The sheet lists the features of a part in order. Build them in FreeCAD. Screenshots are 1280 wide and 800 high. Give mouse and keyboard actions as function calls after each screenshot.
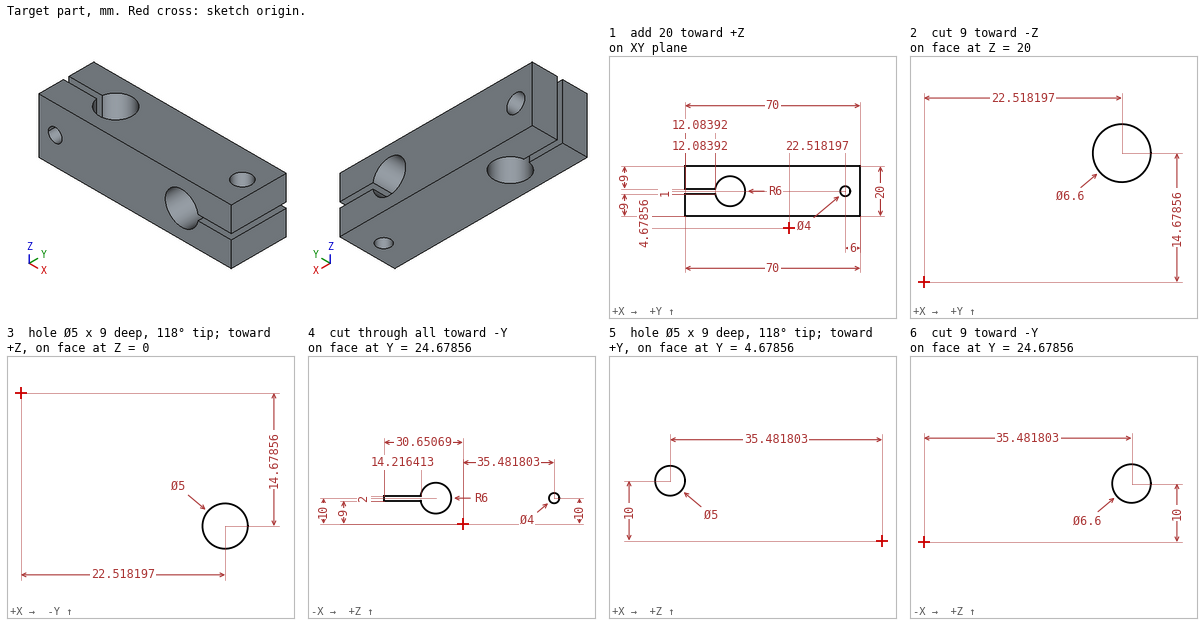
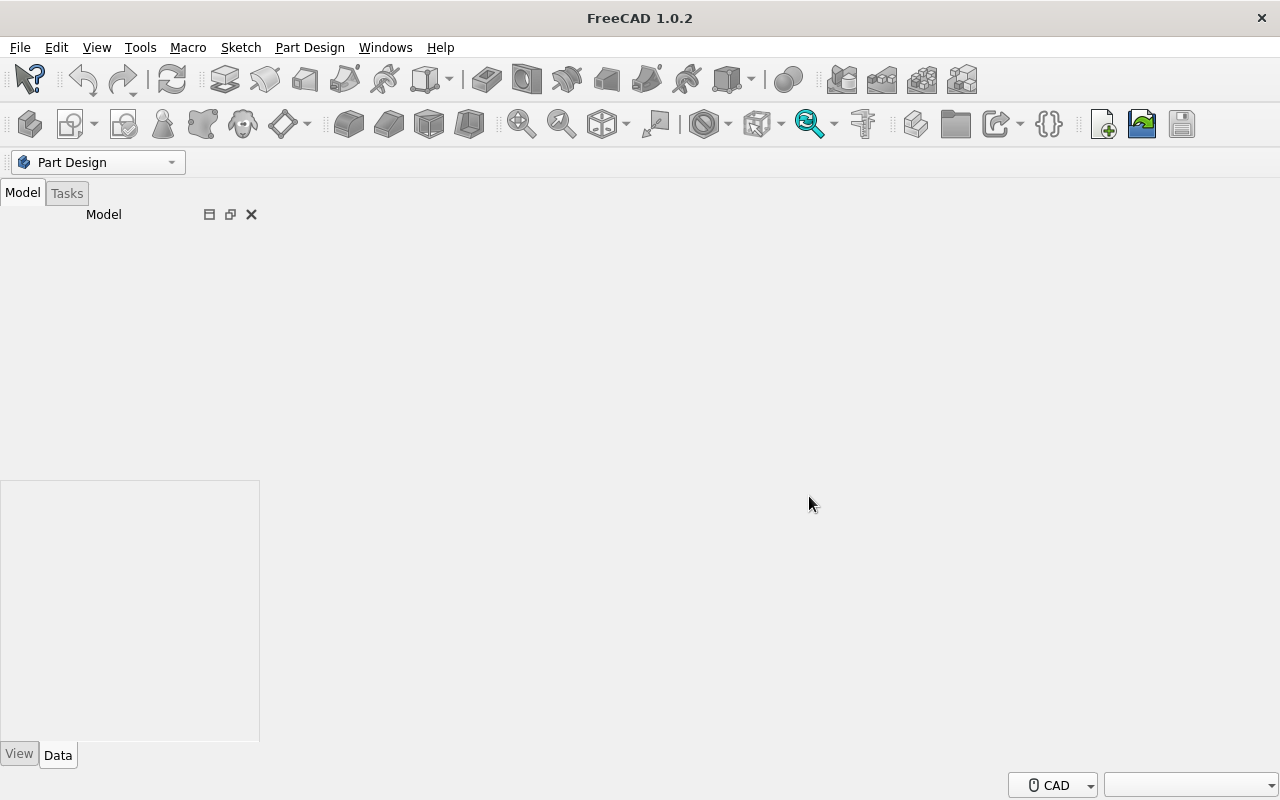
click(1102, 124)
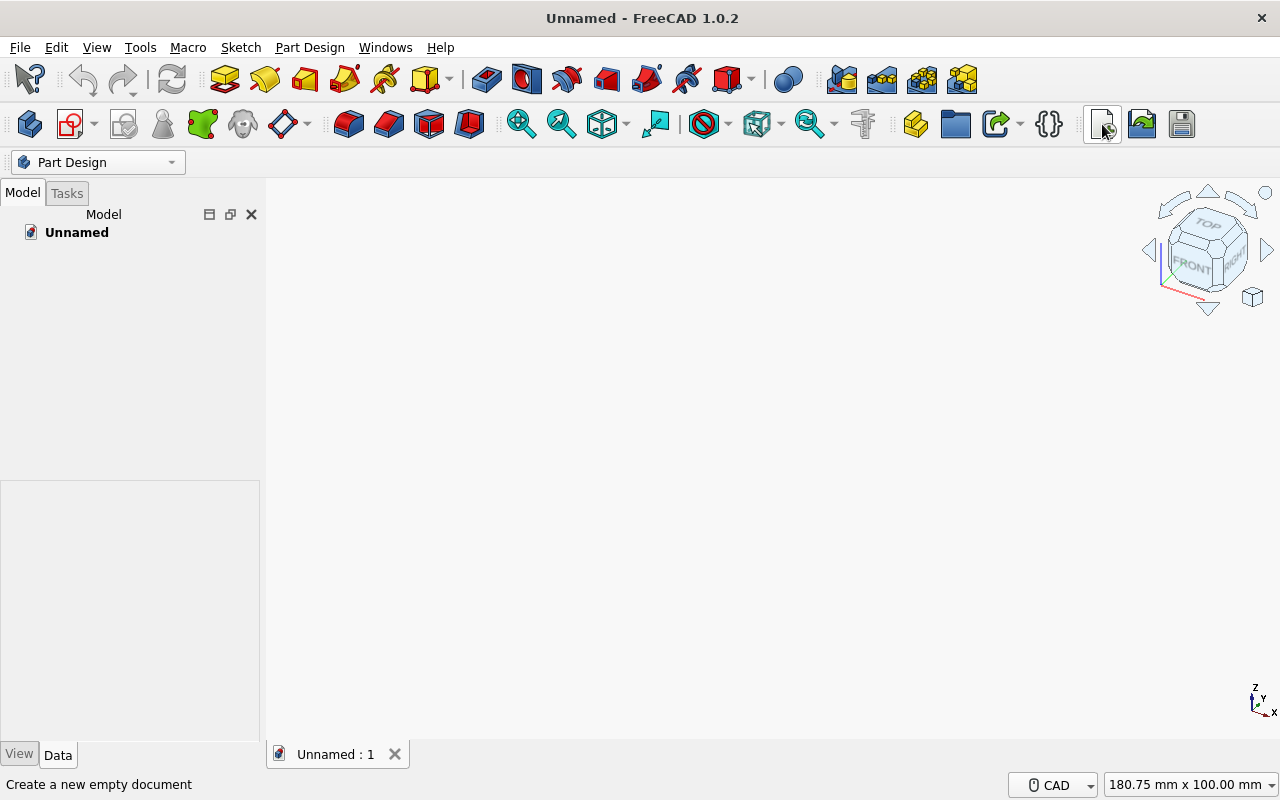
click(70, 124)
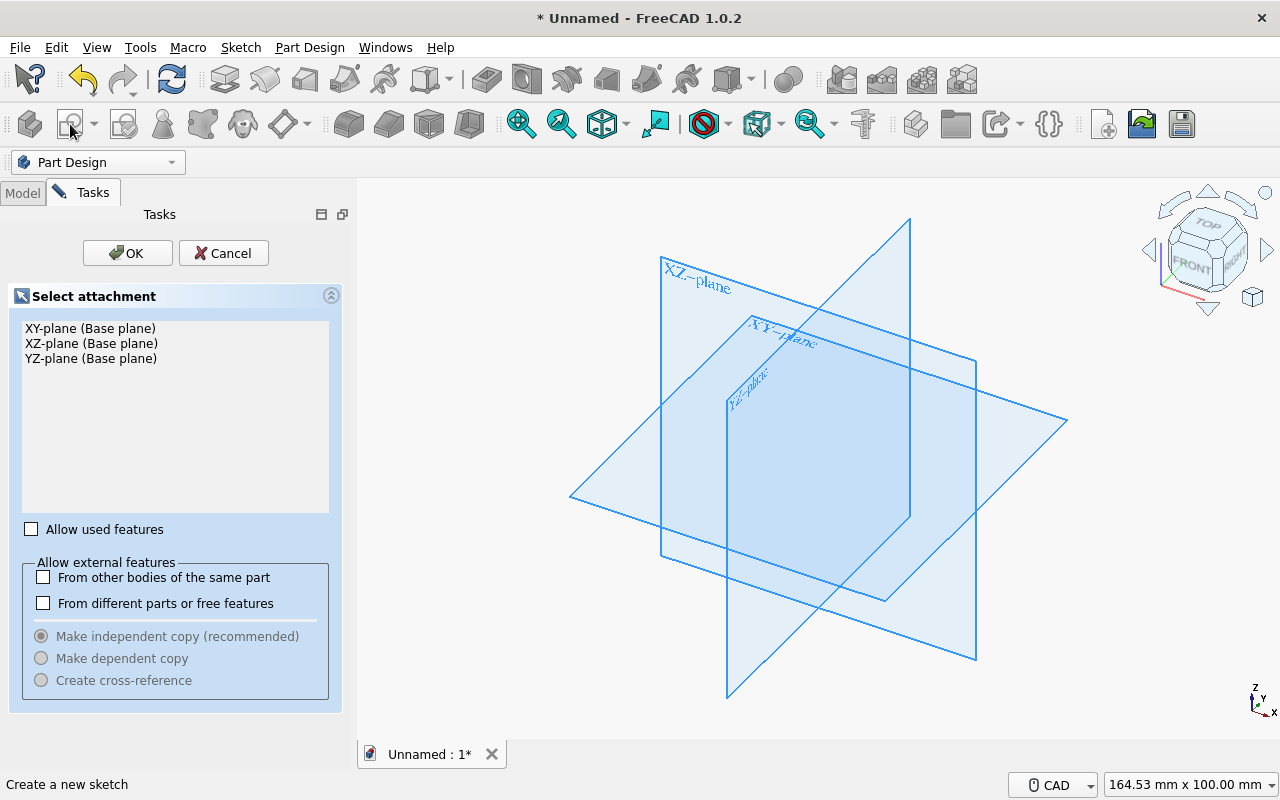
click(82, 328)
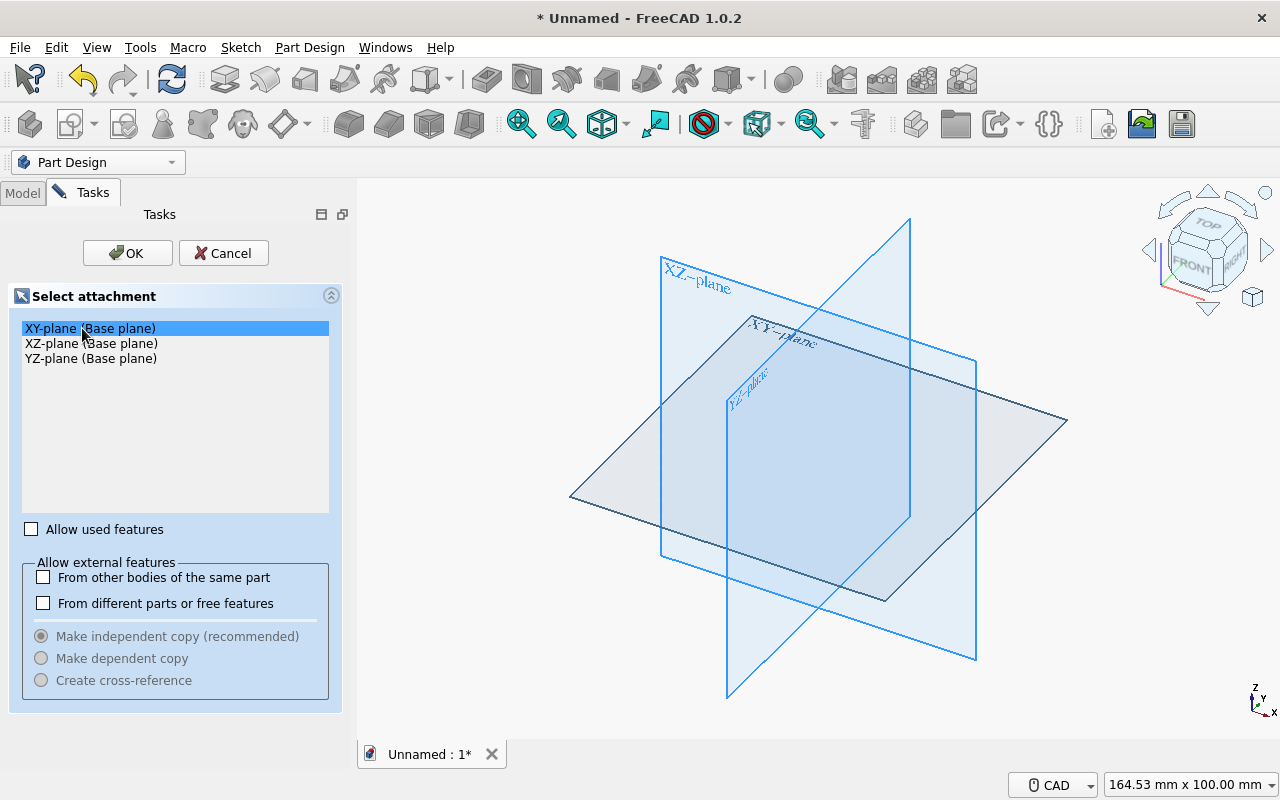
click(128, 253)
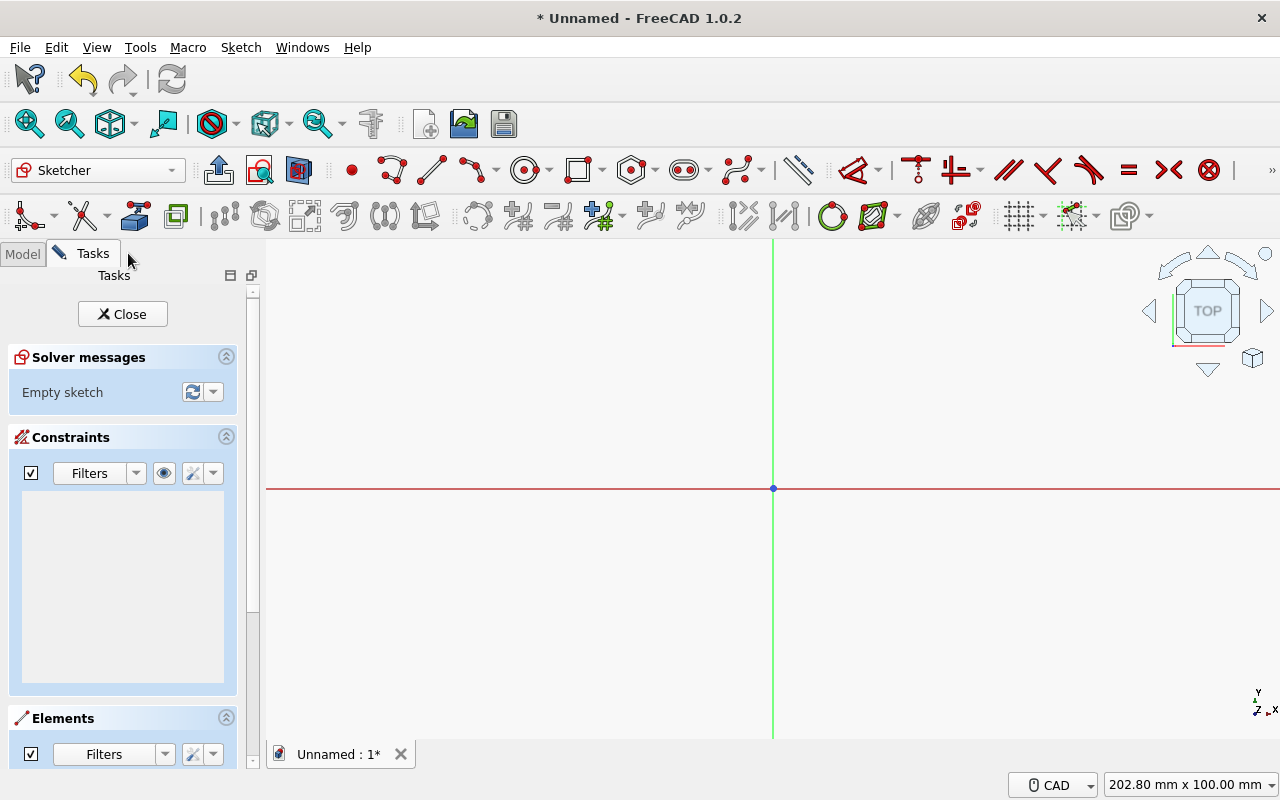
scroll(784, 352, up, 3)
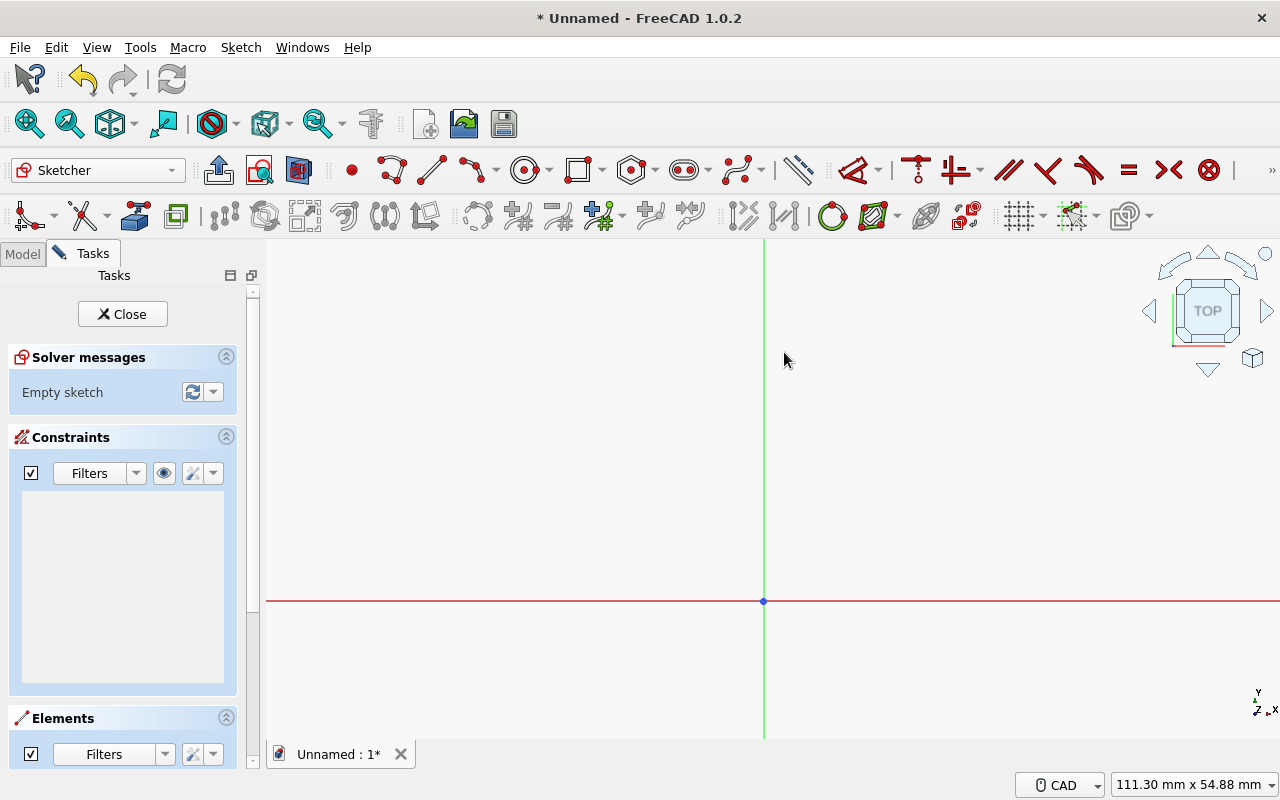
click(392, 170)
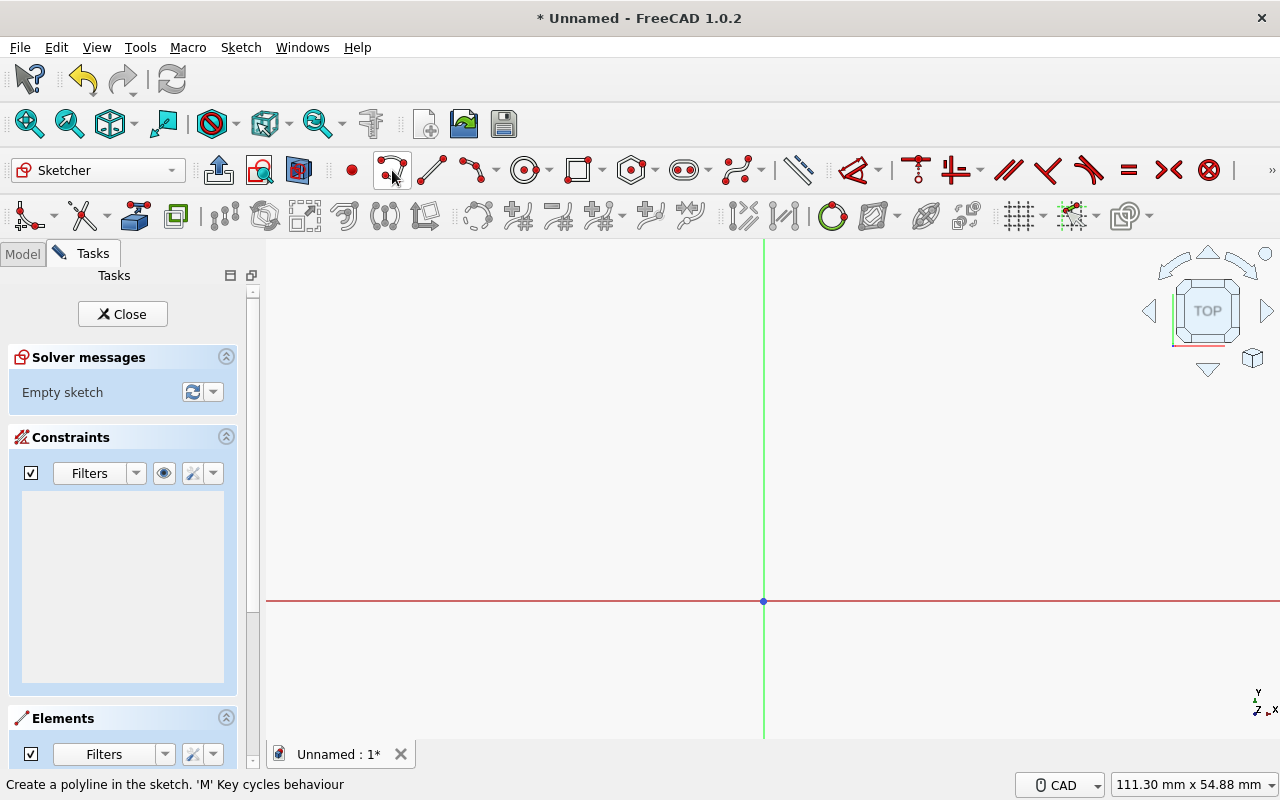
click(496, 477)
click(386, 477)
click(386, 559)
click(1023, 559)
click(1023, 377)
click(386, 377)
click(386, 459)
click(496, 459)
right_click(496, 459)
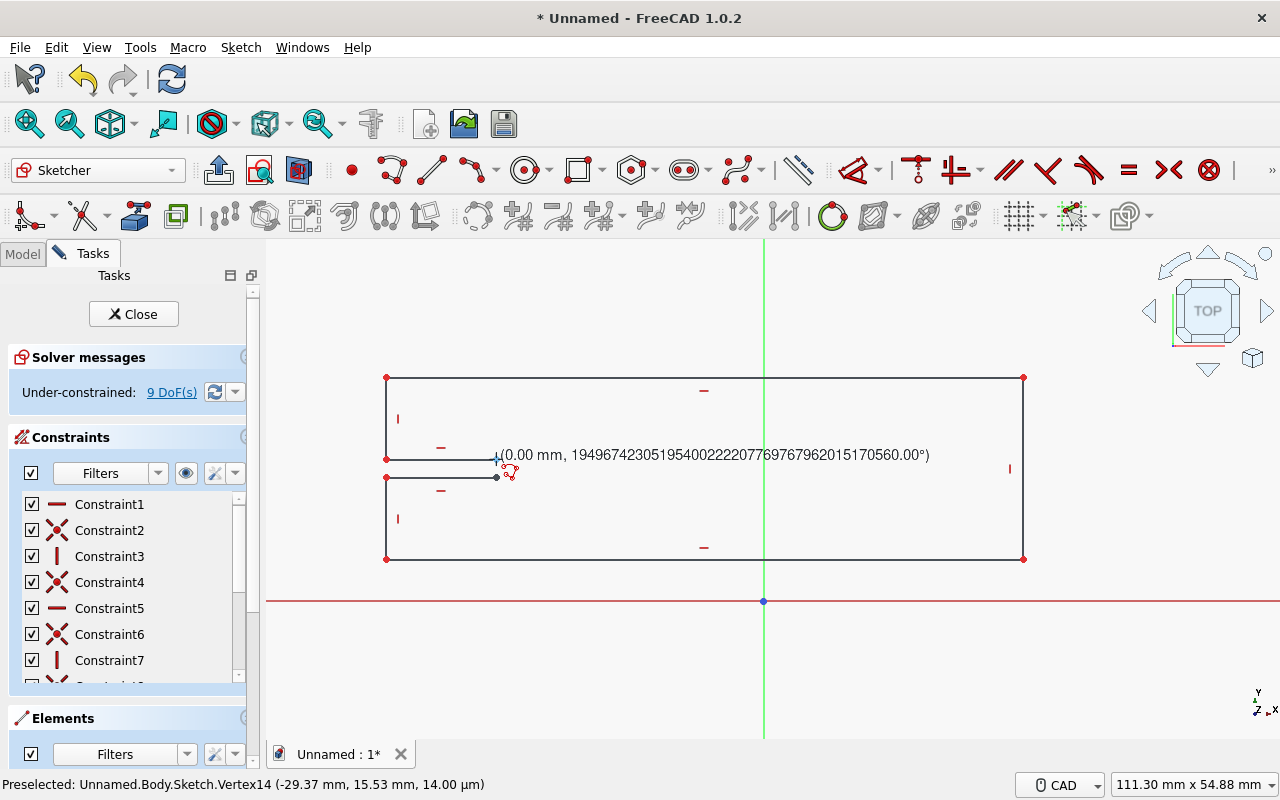
click(472, 170)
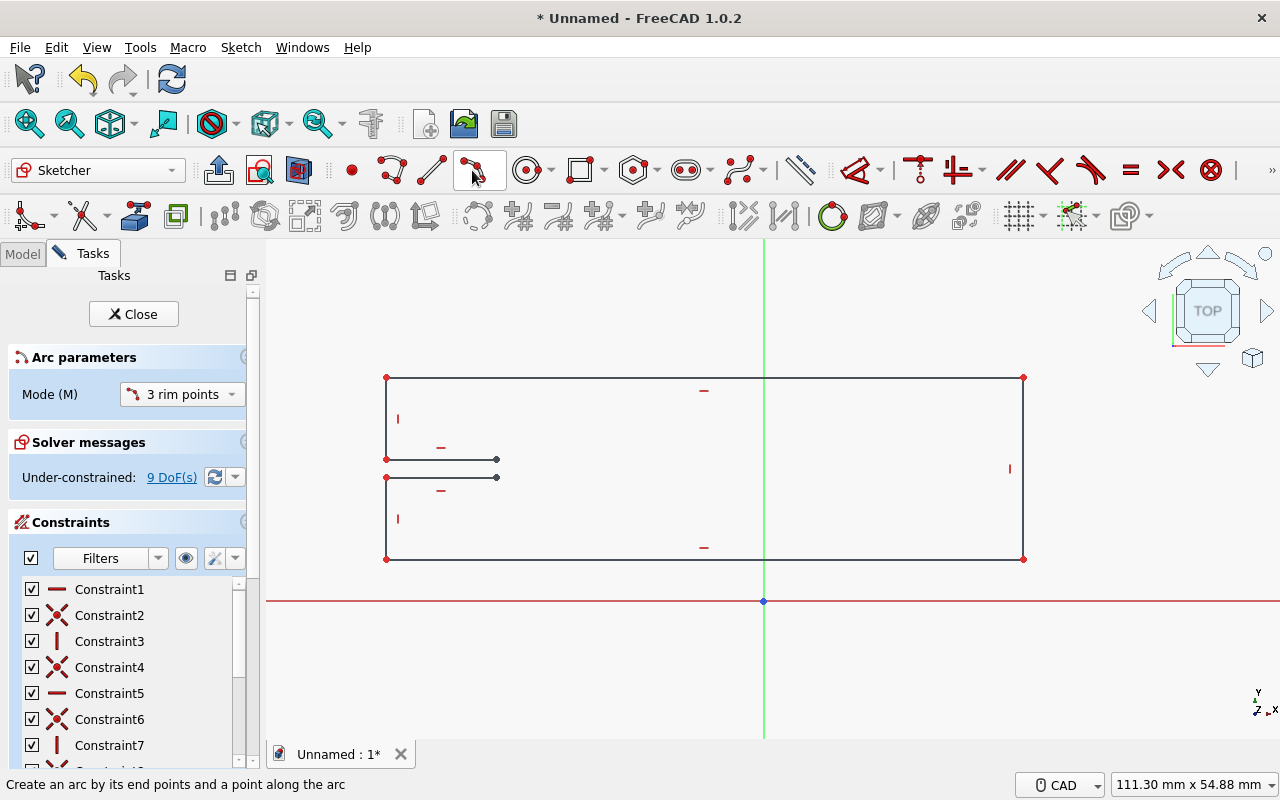
click(496, 460)
click(496, 478)
click(604, 468)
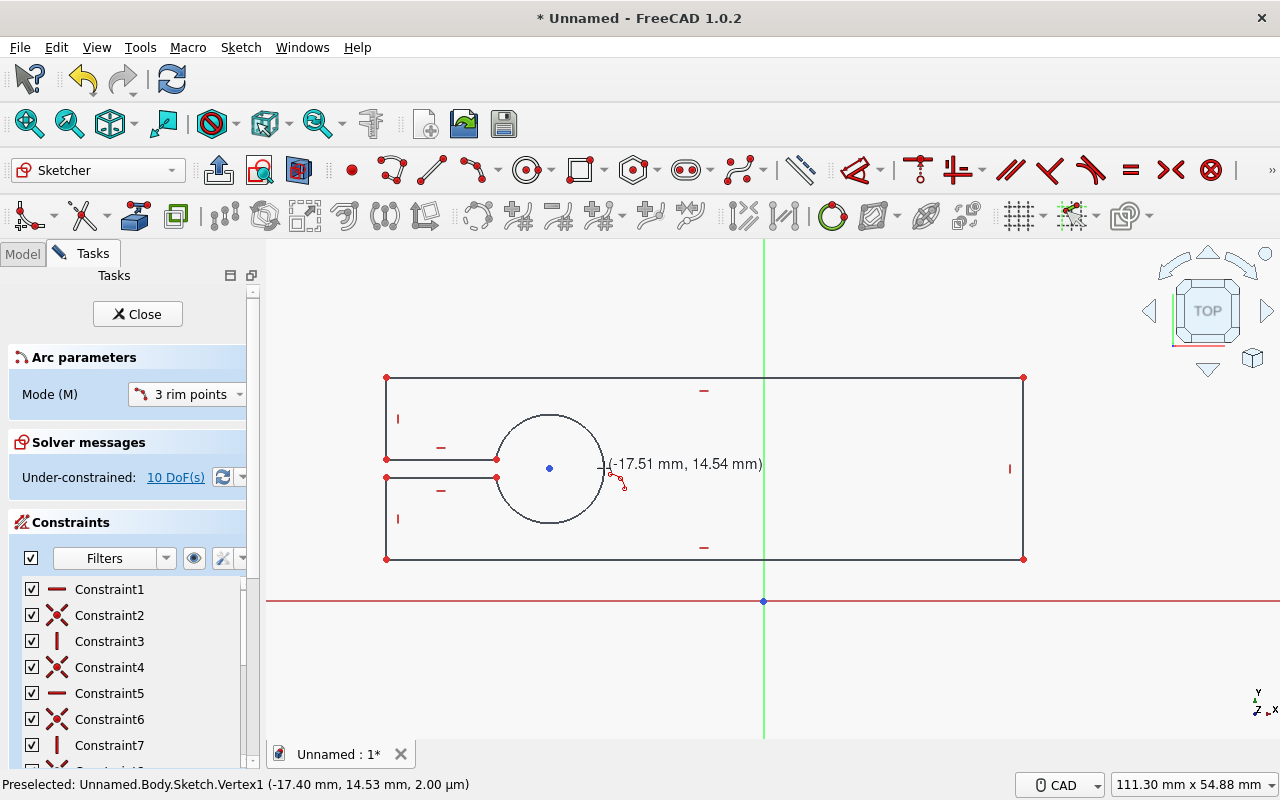
click(528, 170)